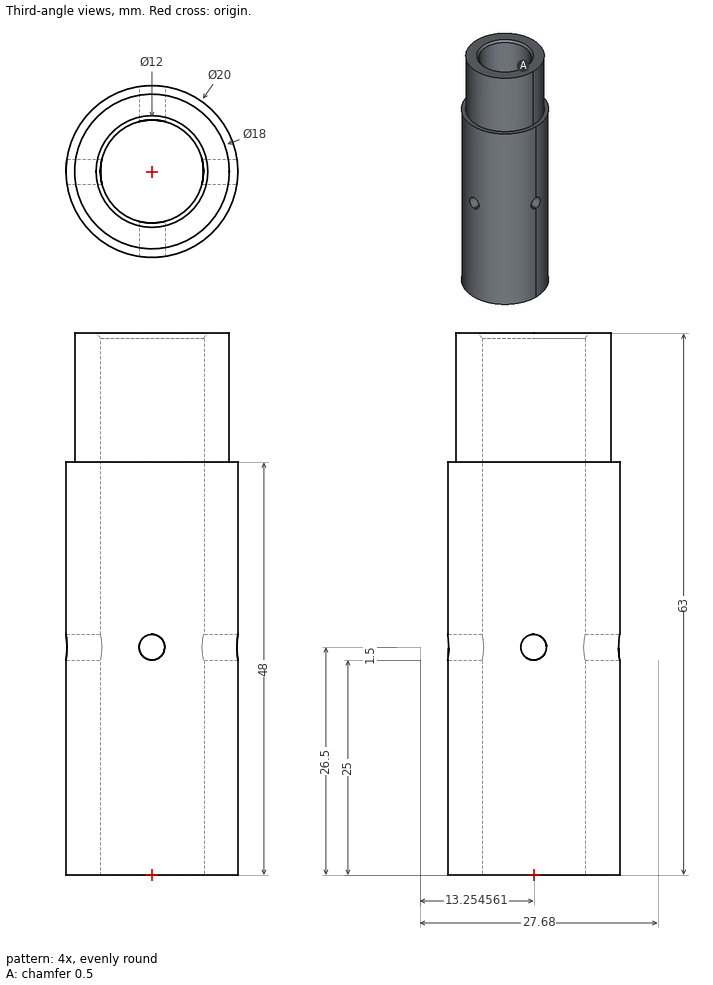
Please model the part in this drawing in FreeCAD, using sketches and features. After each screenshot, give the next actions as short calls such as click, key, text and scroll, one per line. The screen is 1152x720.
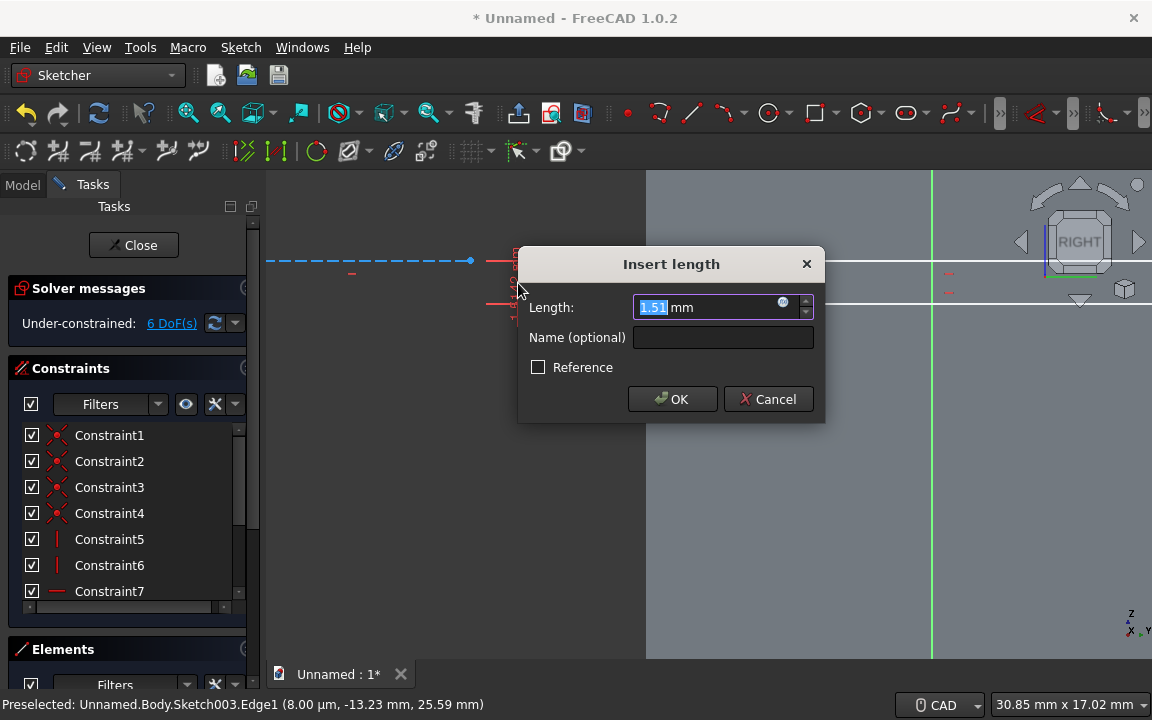
text(1.5)
key(Return)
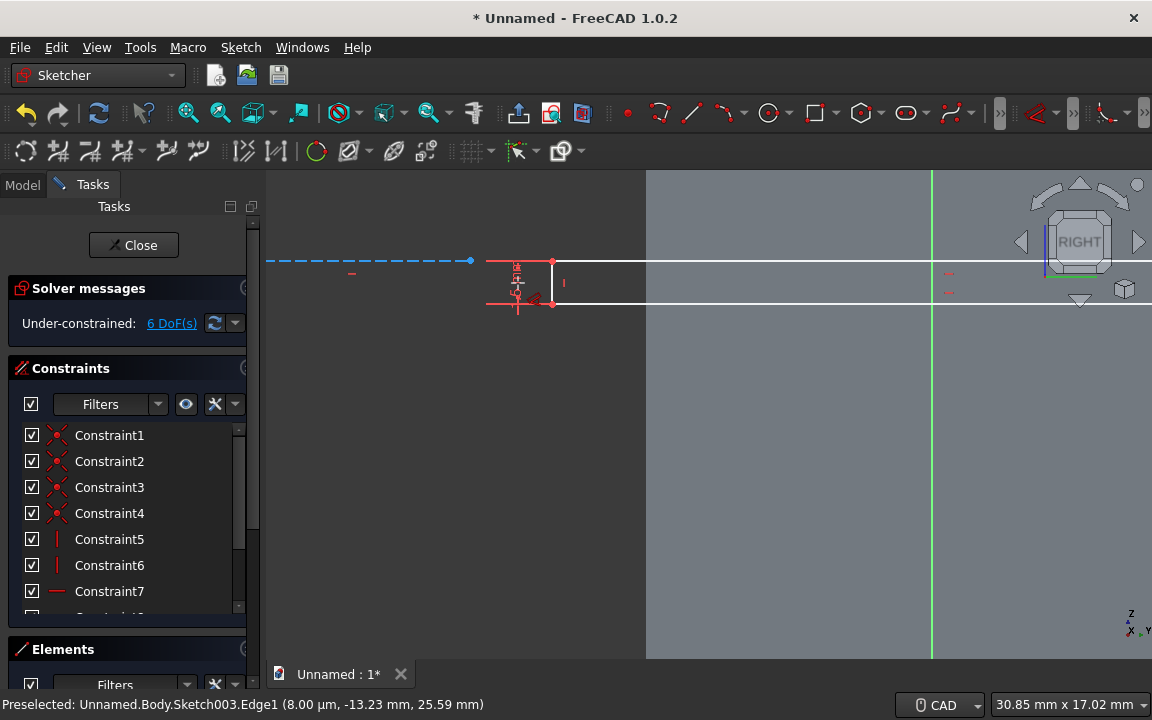
click(552, 304)
click(518, 468)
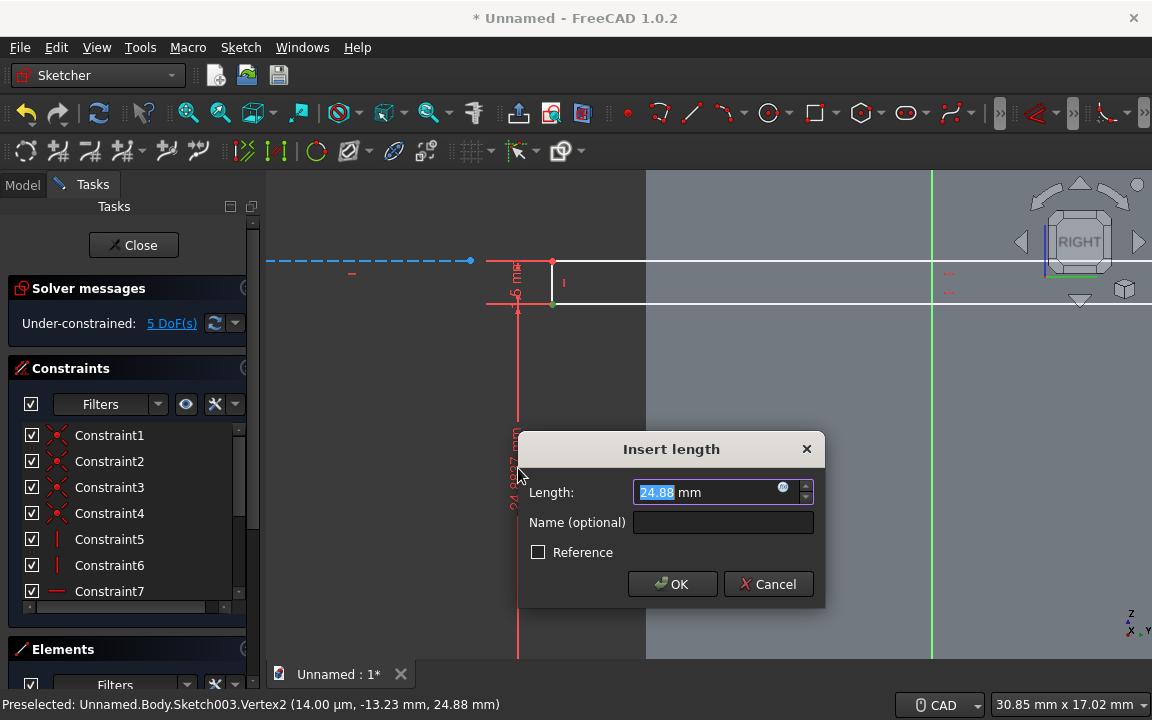
text(25)
key(Return)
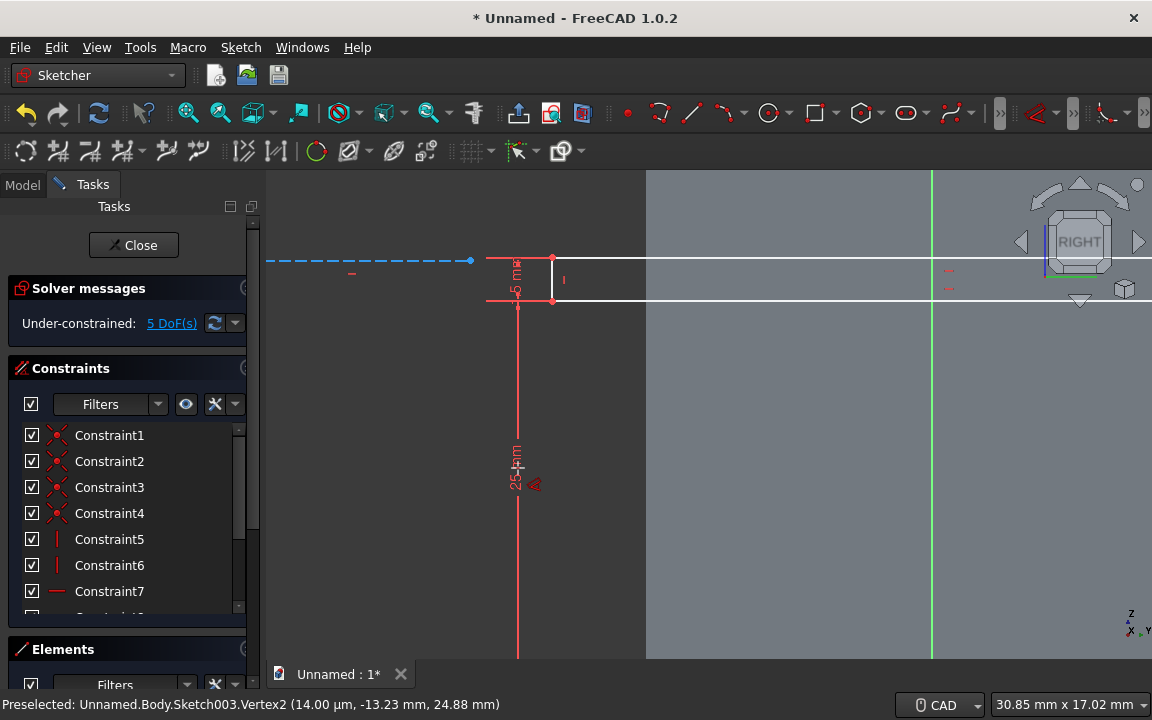
click(791, 301)
click(770, 335)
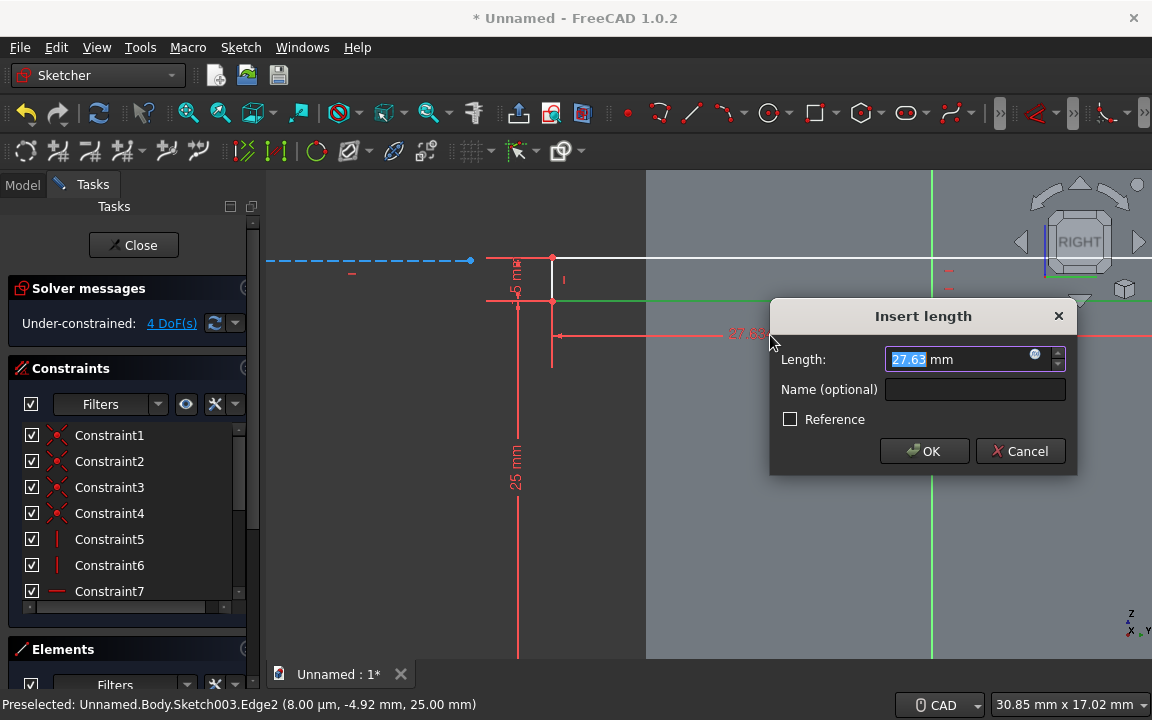
text(27.68)
key(Return)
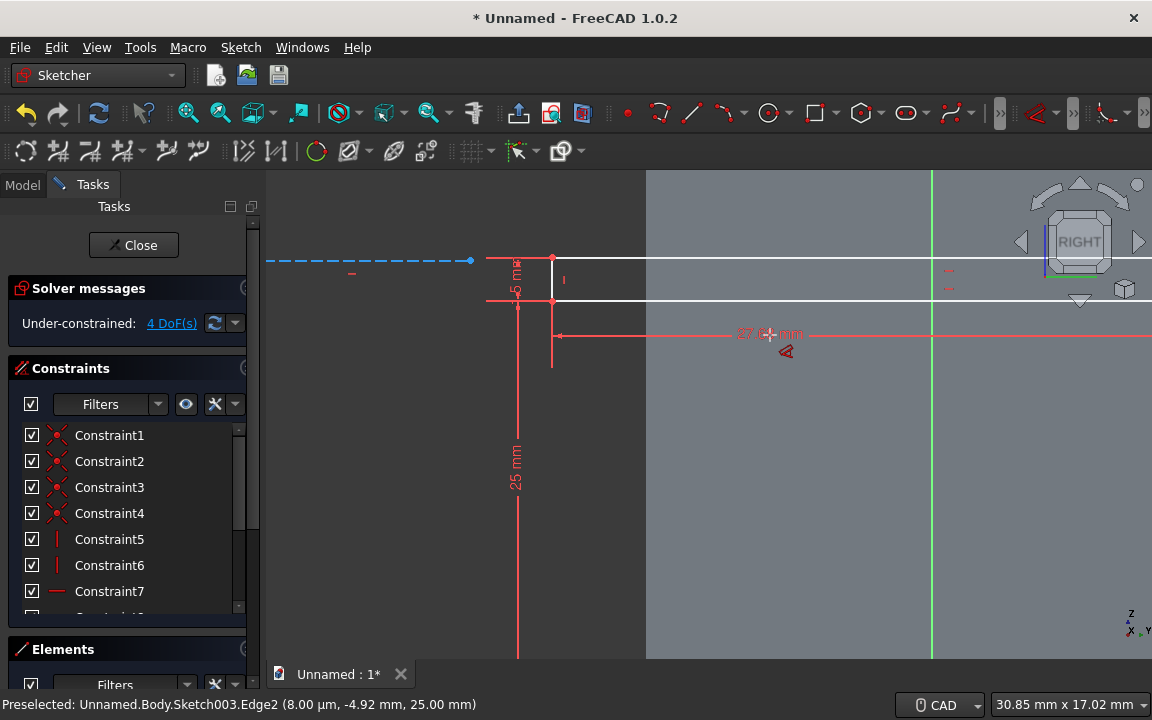
click(471, 261)
click(437, 446)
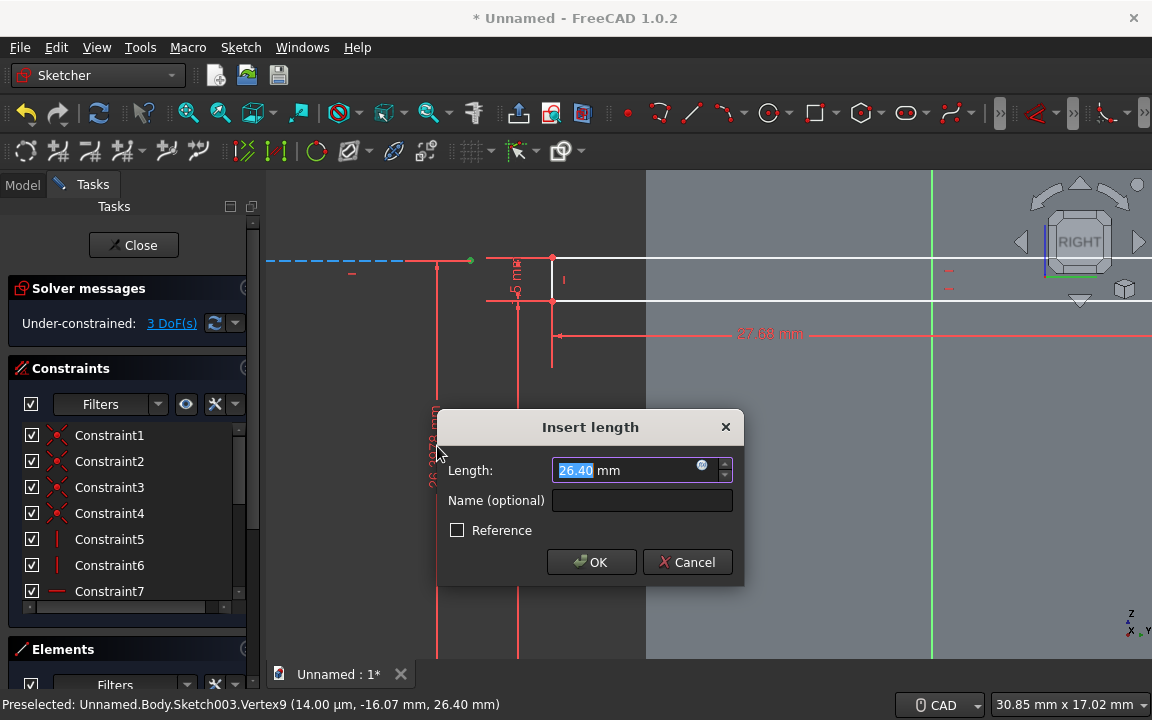
text(26.5)
key(Return)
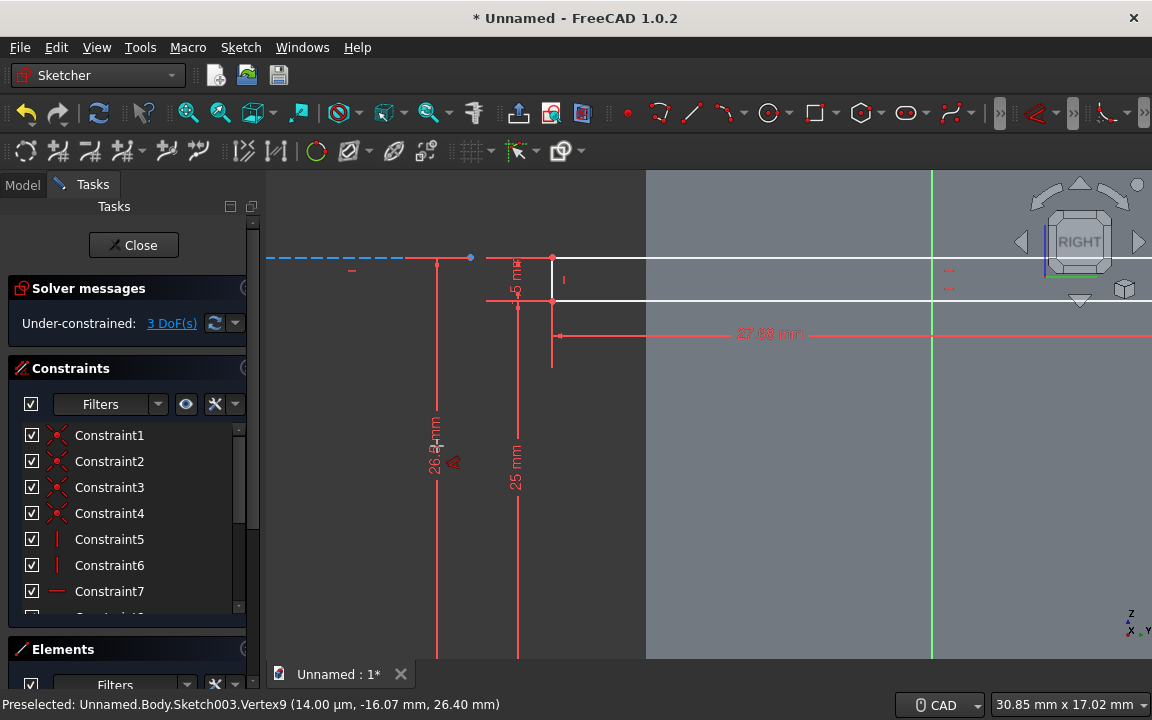
click(552, 258)
click(742, 224)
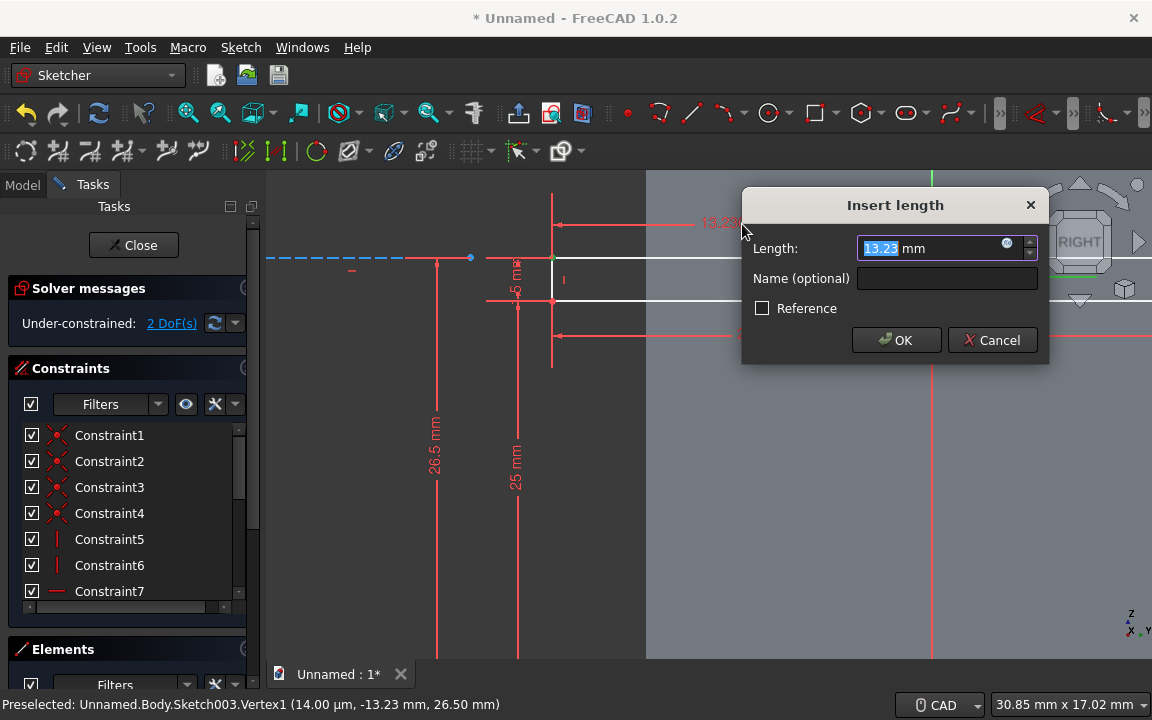
text(13.254561)
key(Return)
key(Escape)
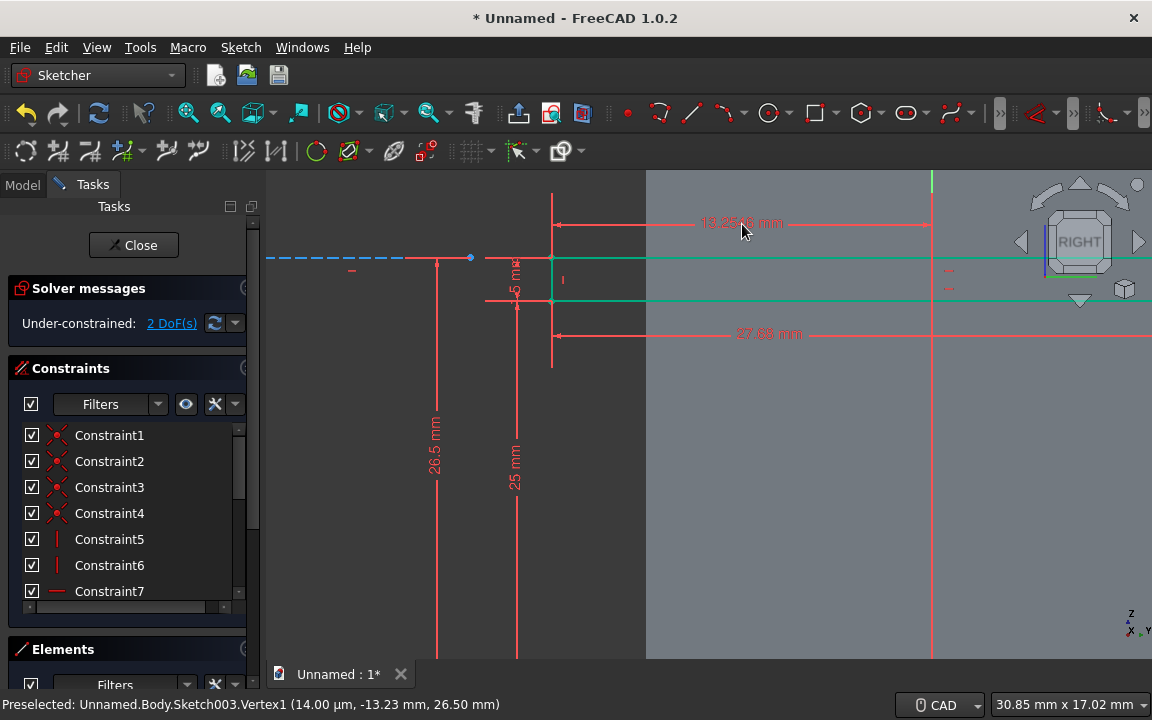
click(134, 245)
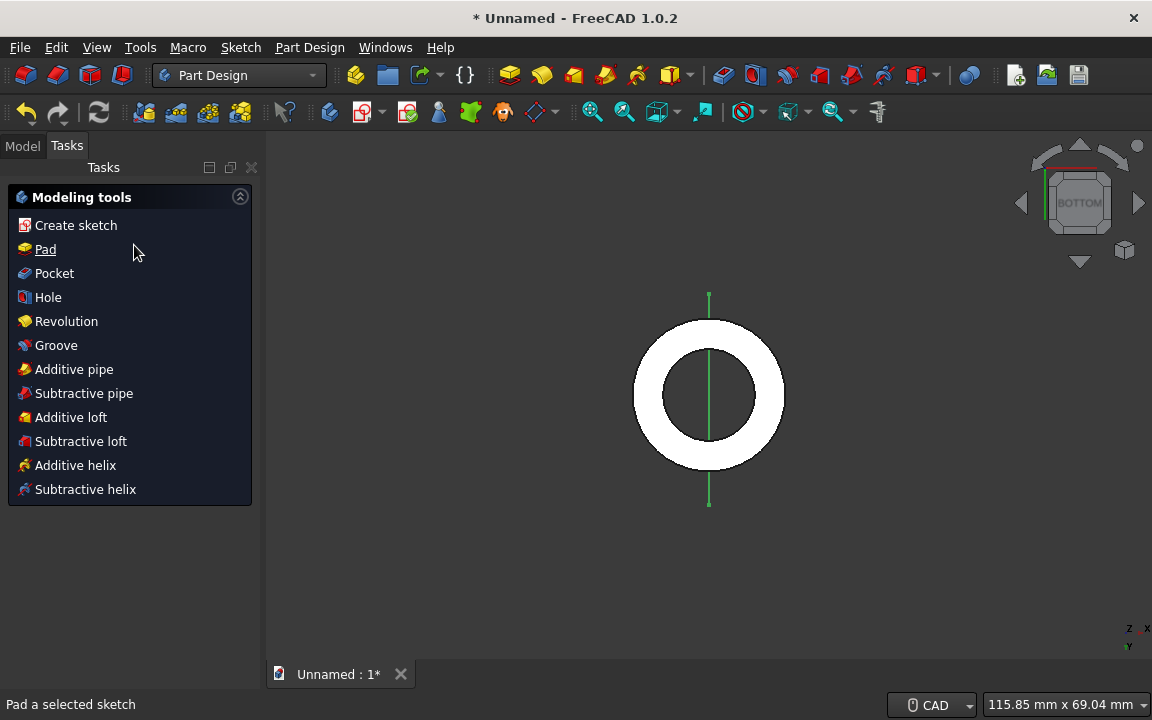
click(788, 76)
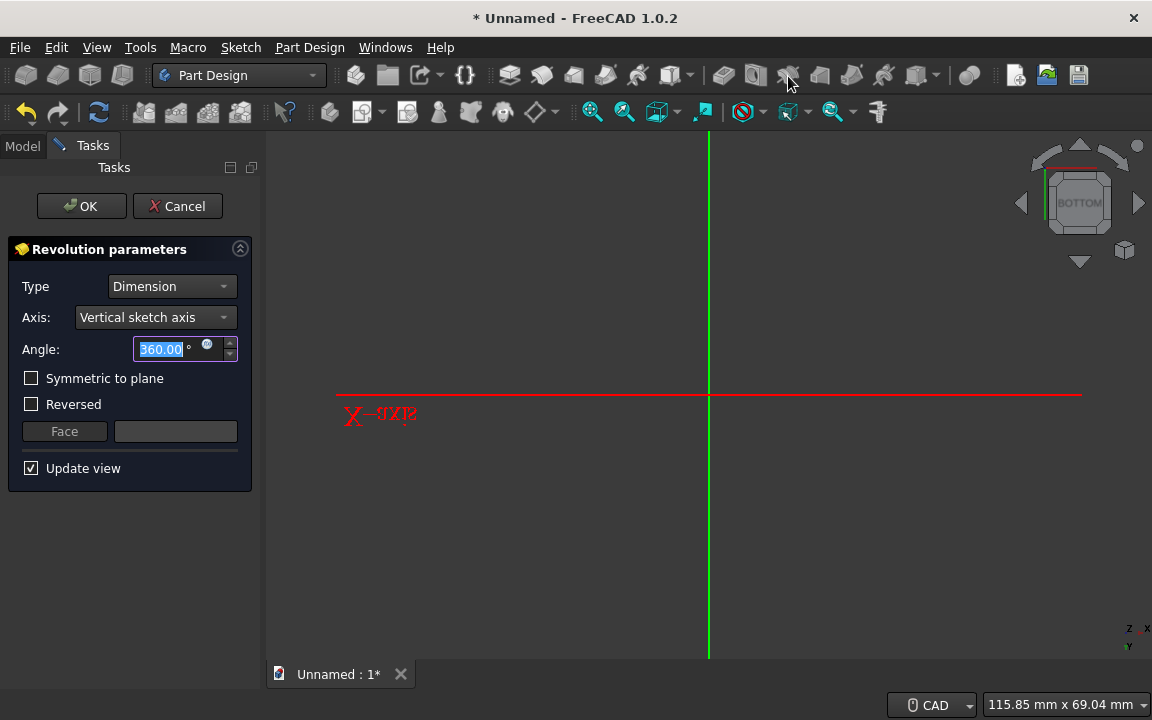
click(156, 318)